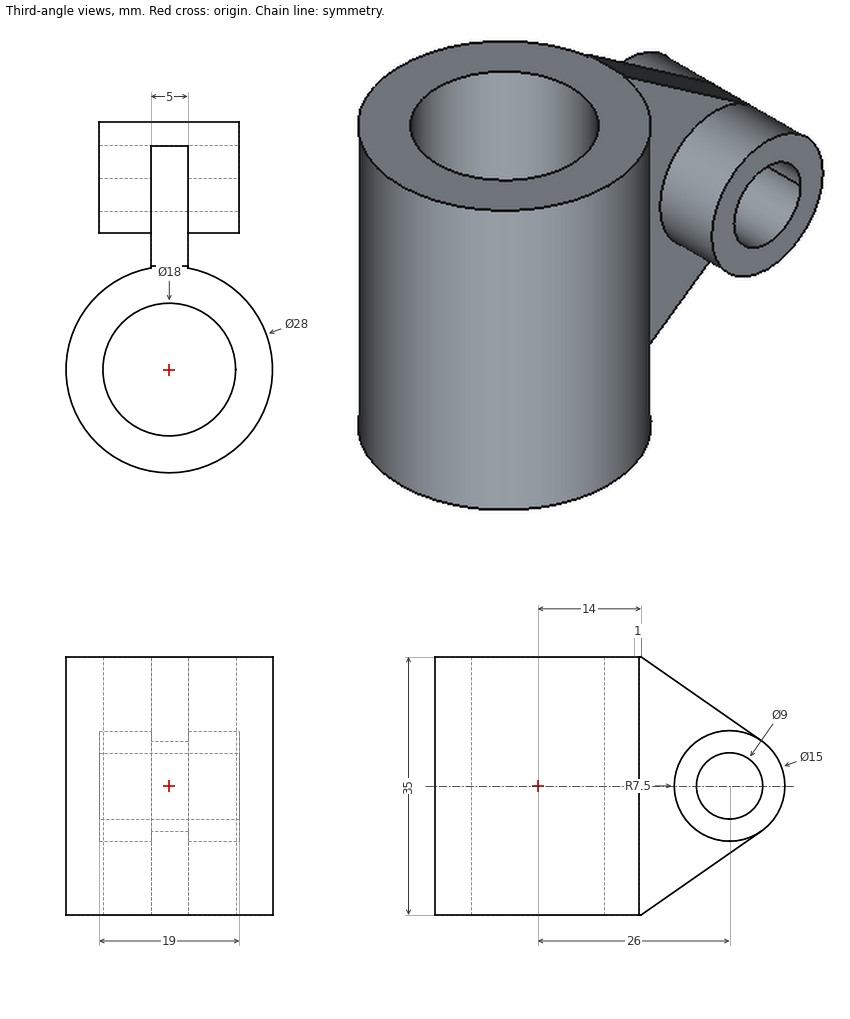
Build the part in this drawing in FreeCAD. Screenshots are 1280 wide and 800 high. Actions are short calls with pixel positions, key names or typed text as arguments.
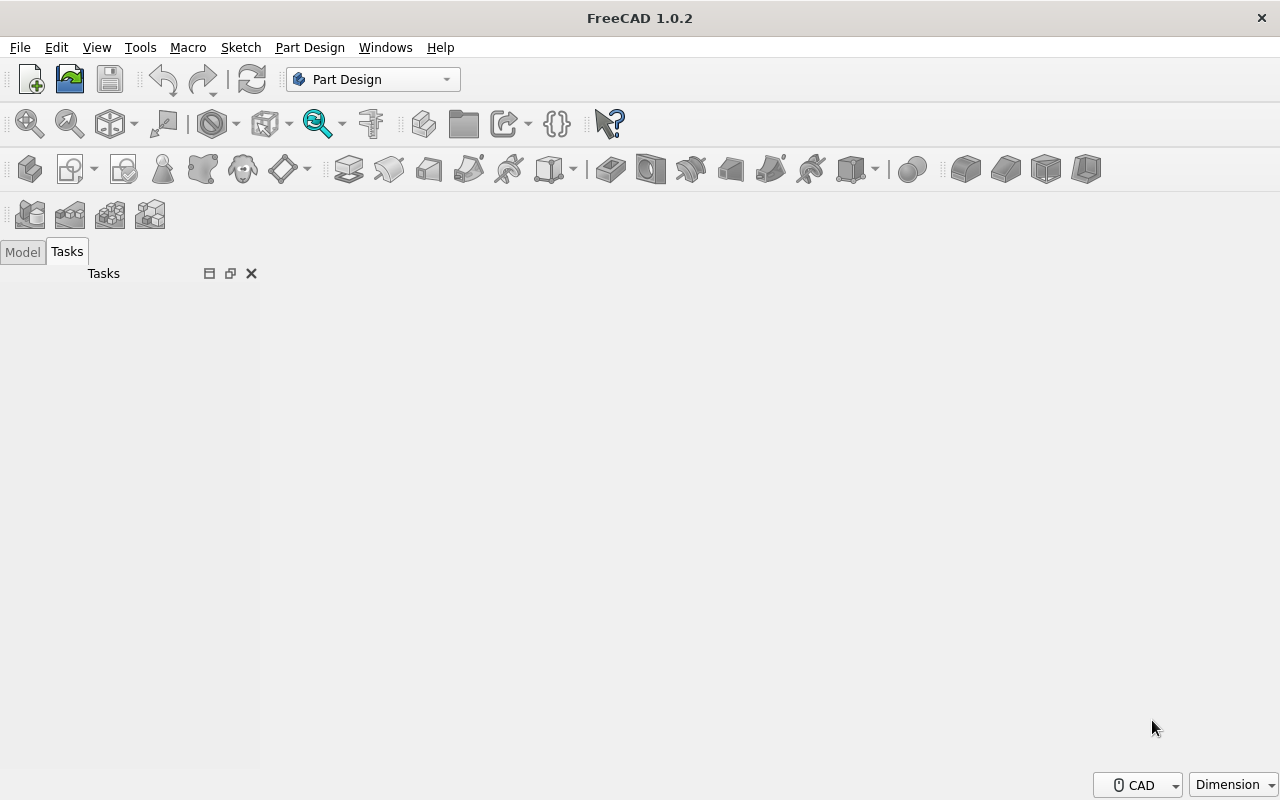
click(30, 80)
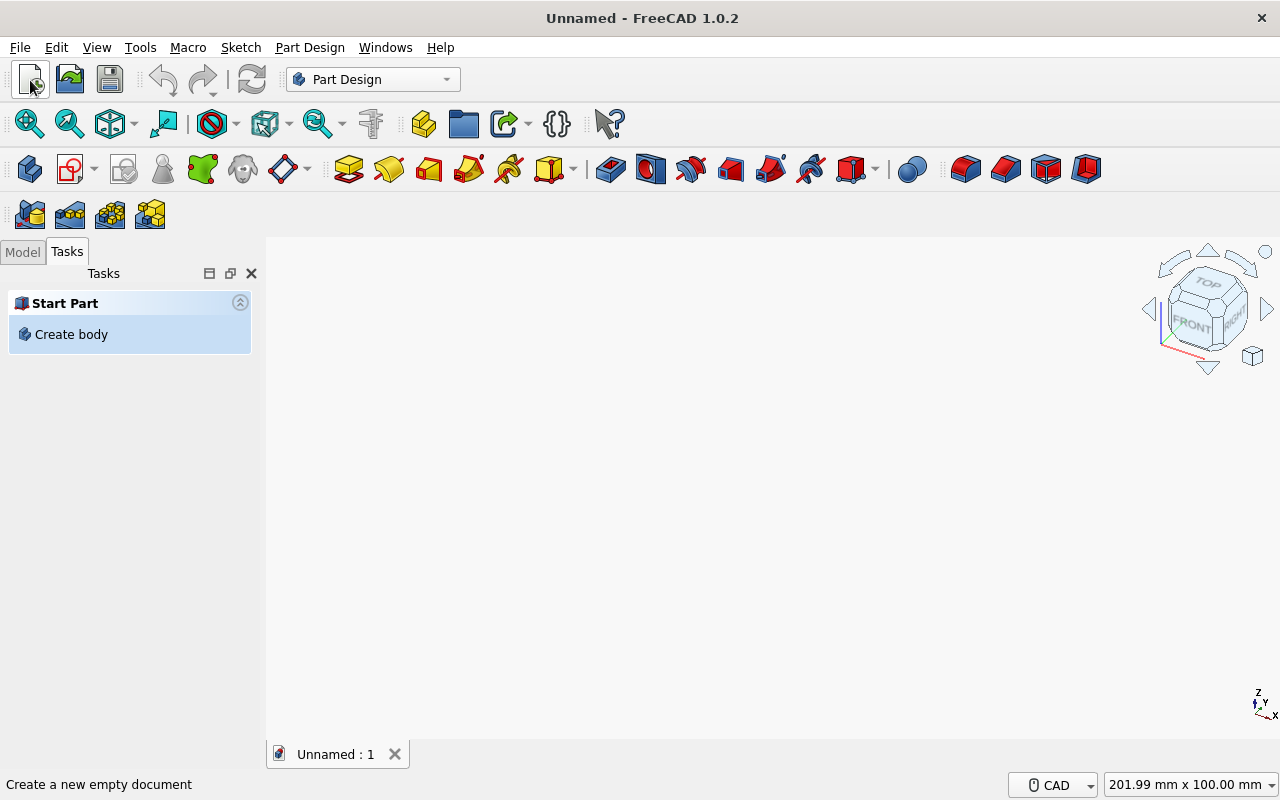
click(70, 170)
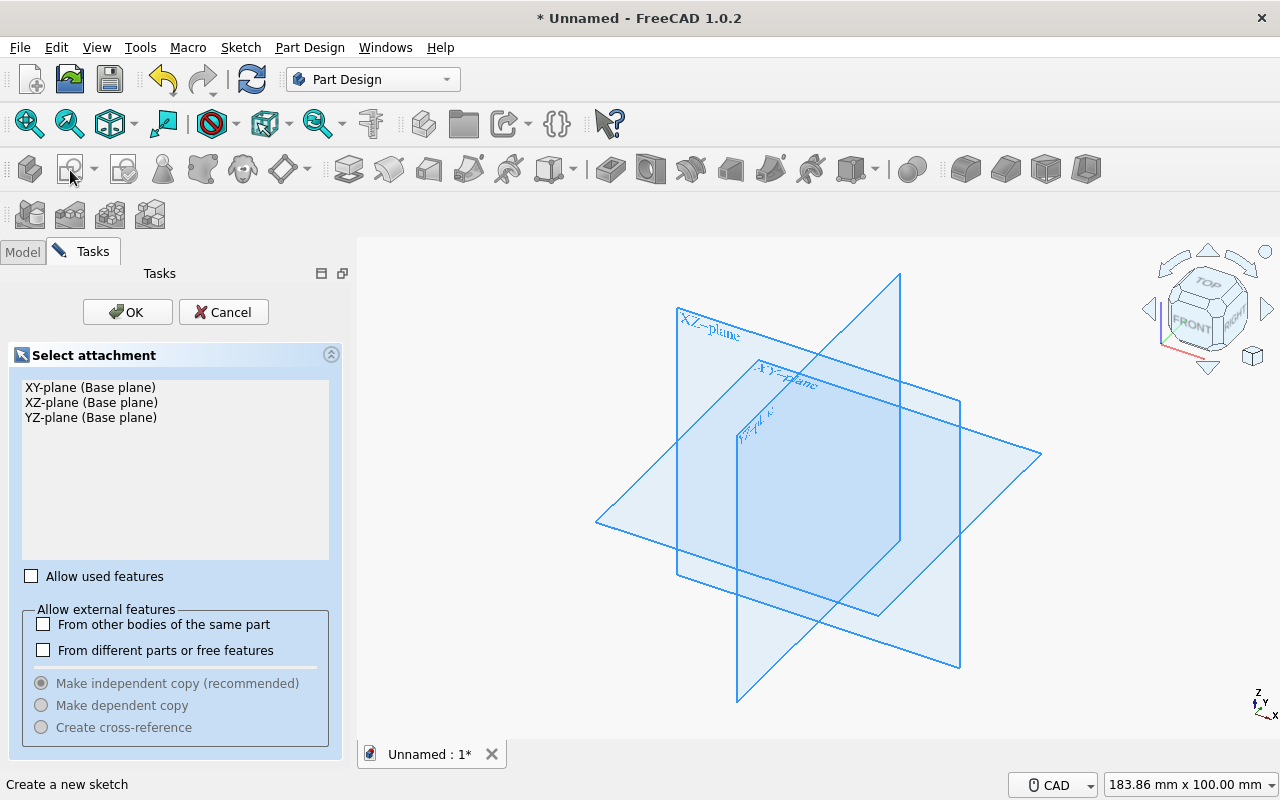
click(82, 388)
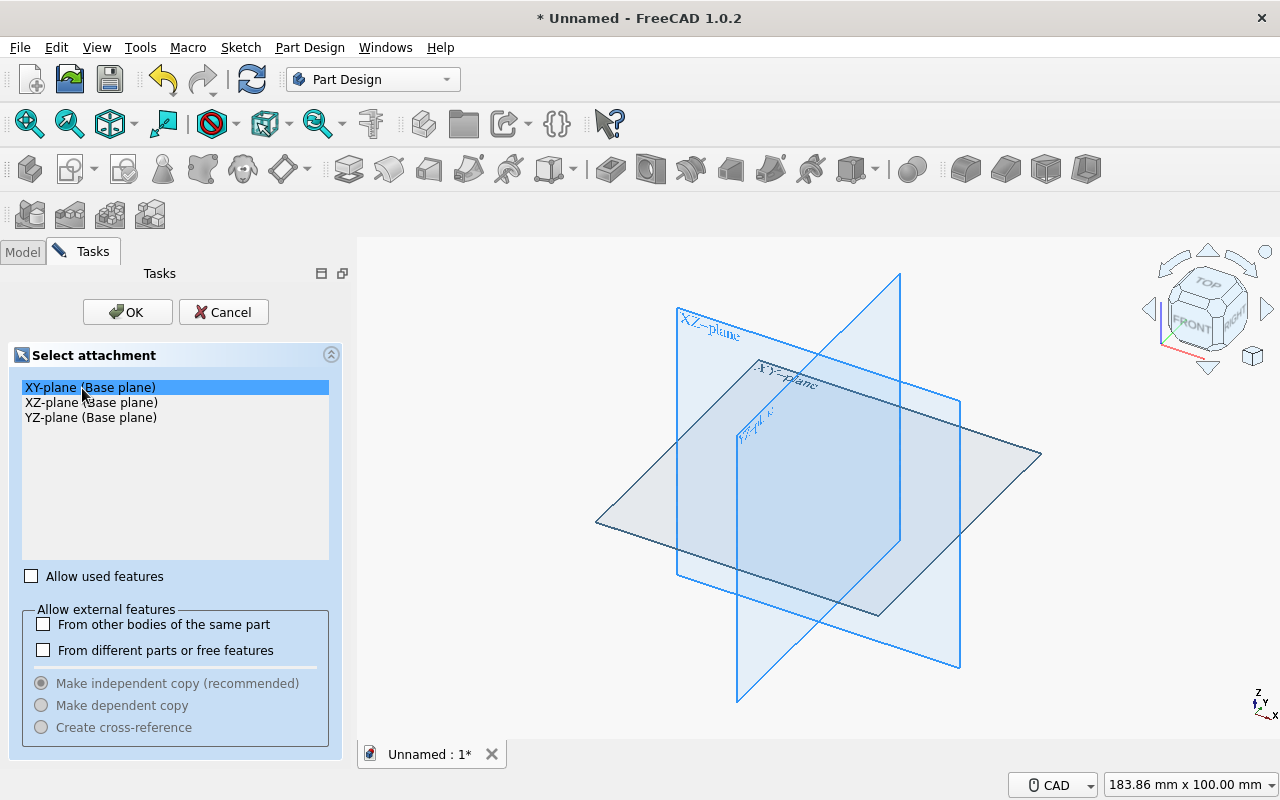
click(128, 312)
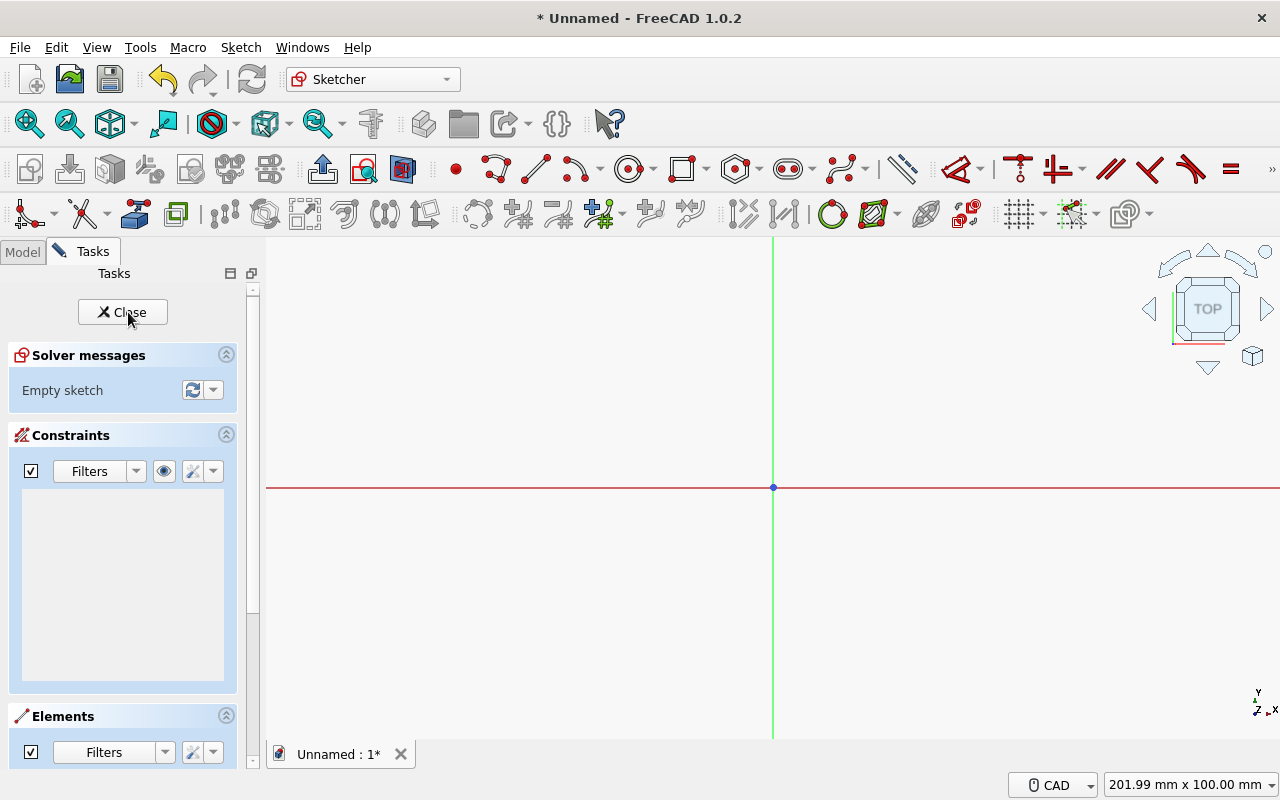
scroll(829, 488, up, 4)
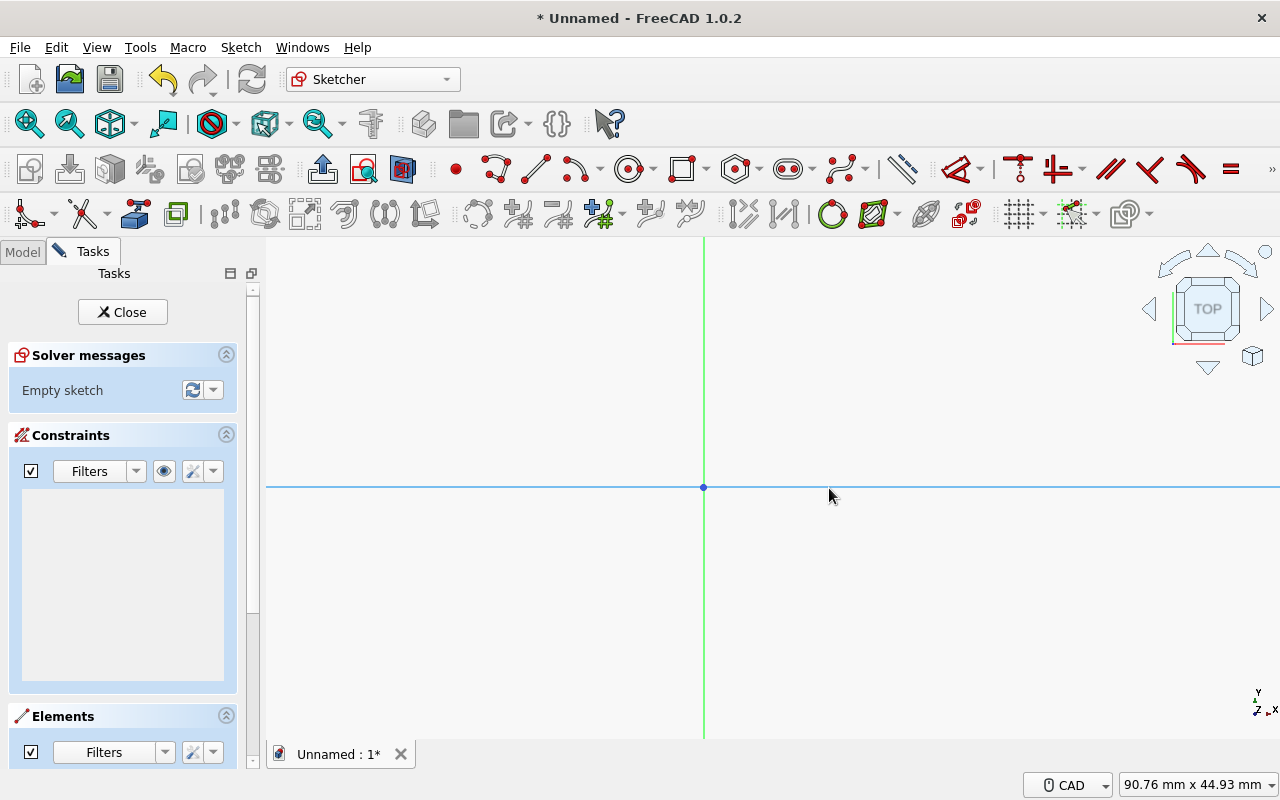
key(g)
key(c)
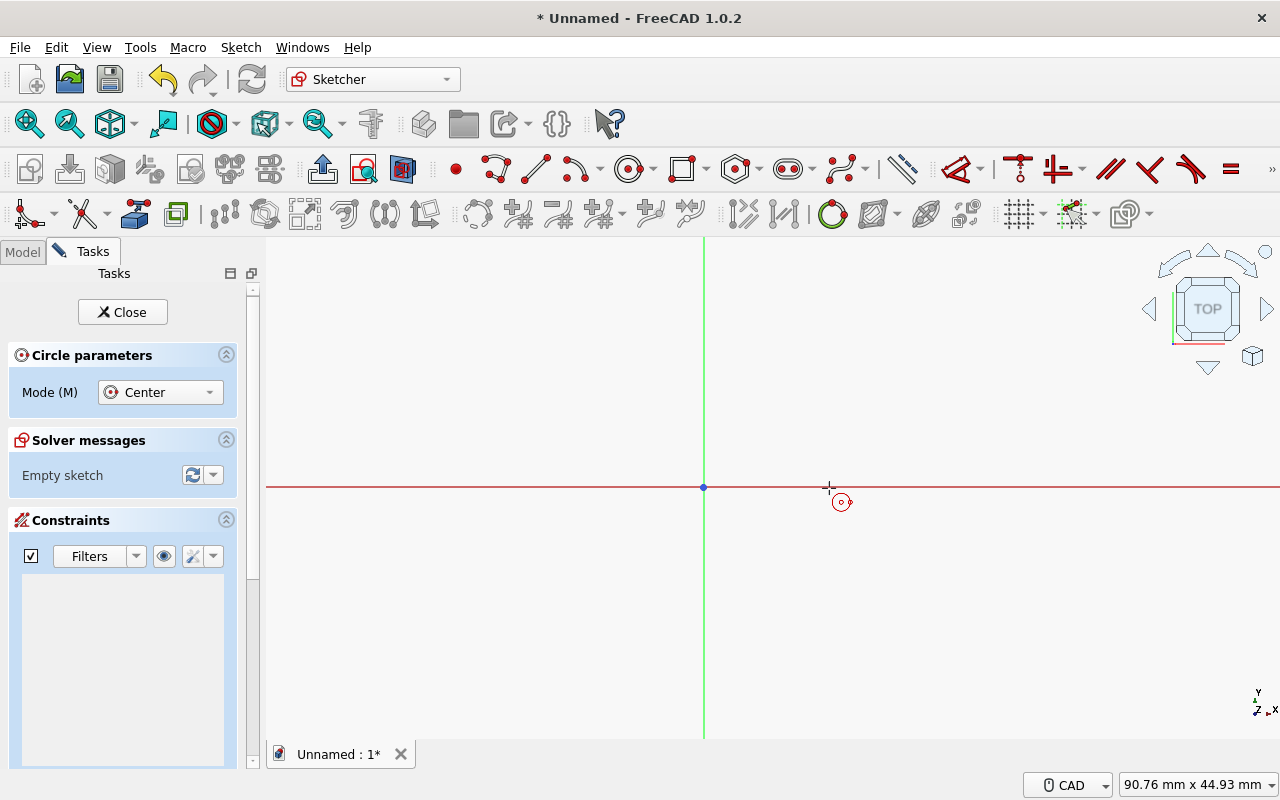
click(704, 487)
click(814, 377)
key(Escape)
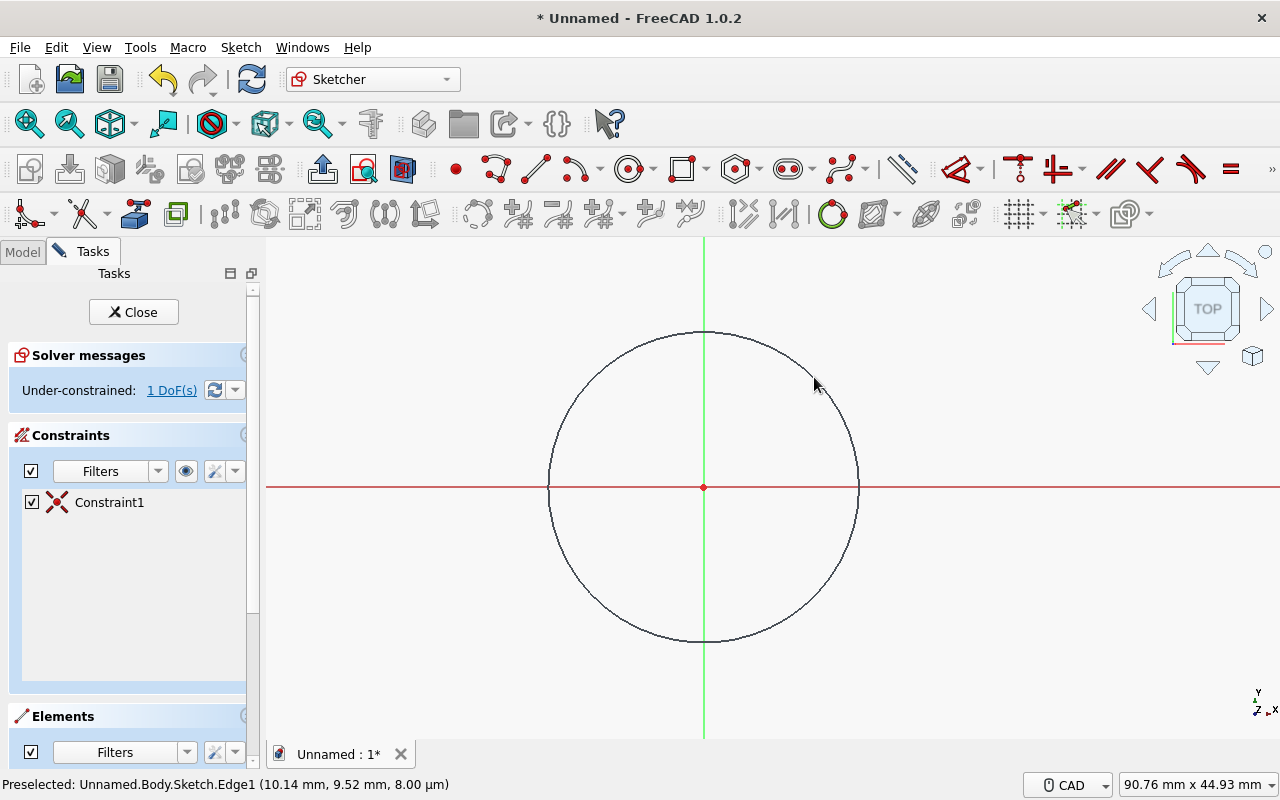
key(d)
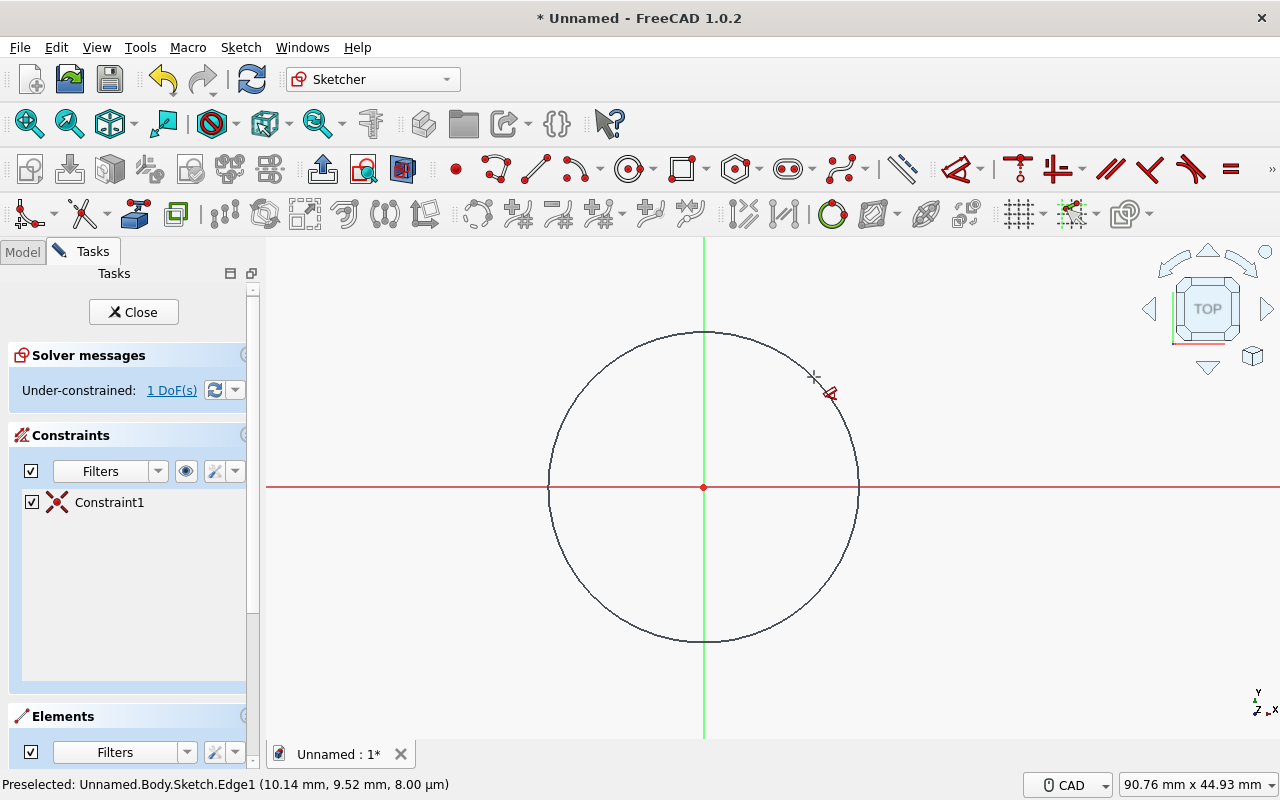
click(813, 377)
click(836, 354)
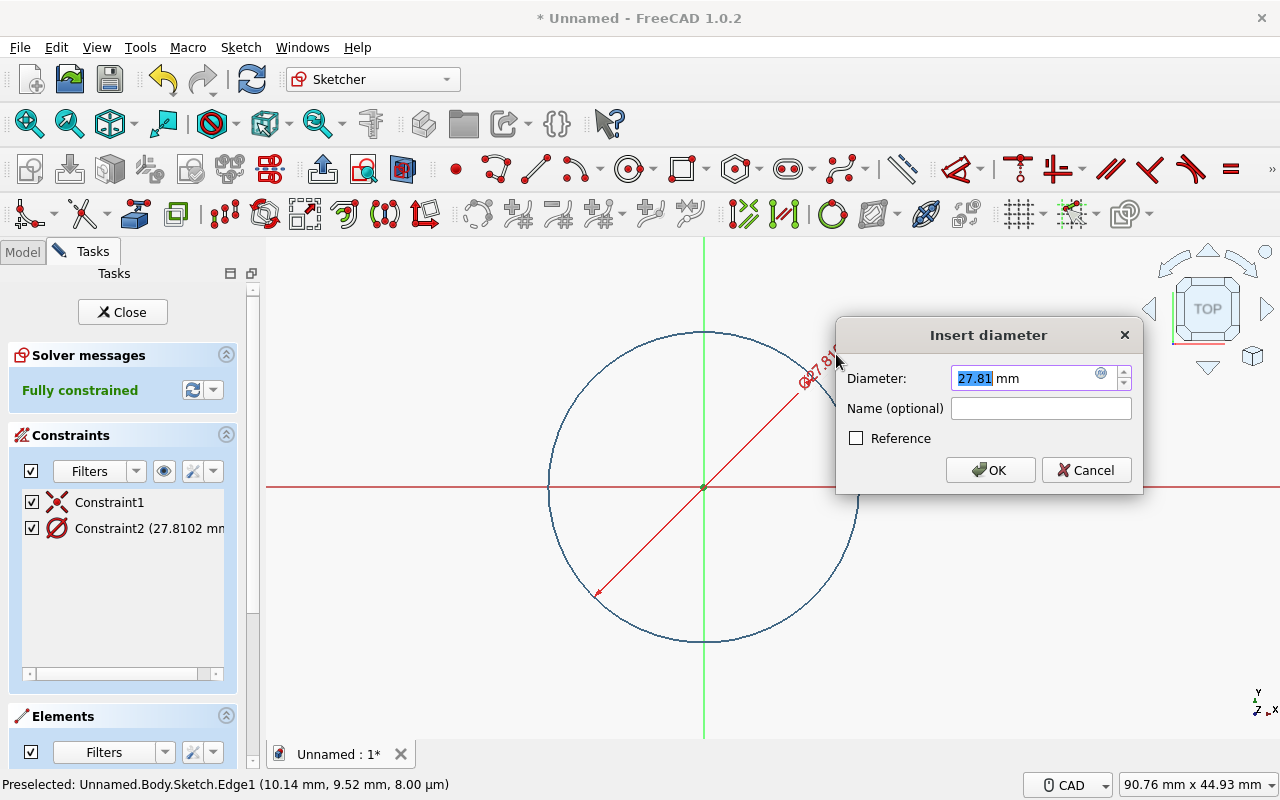
text(28)
key(Return)
key(Escape)